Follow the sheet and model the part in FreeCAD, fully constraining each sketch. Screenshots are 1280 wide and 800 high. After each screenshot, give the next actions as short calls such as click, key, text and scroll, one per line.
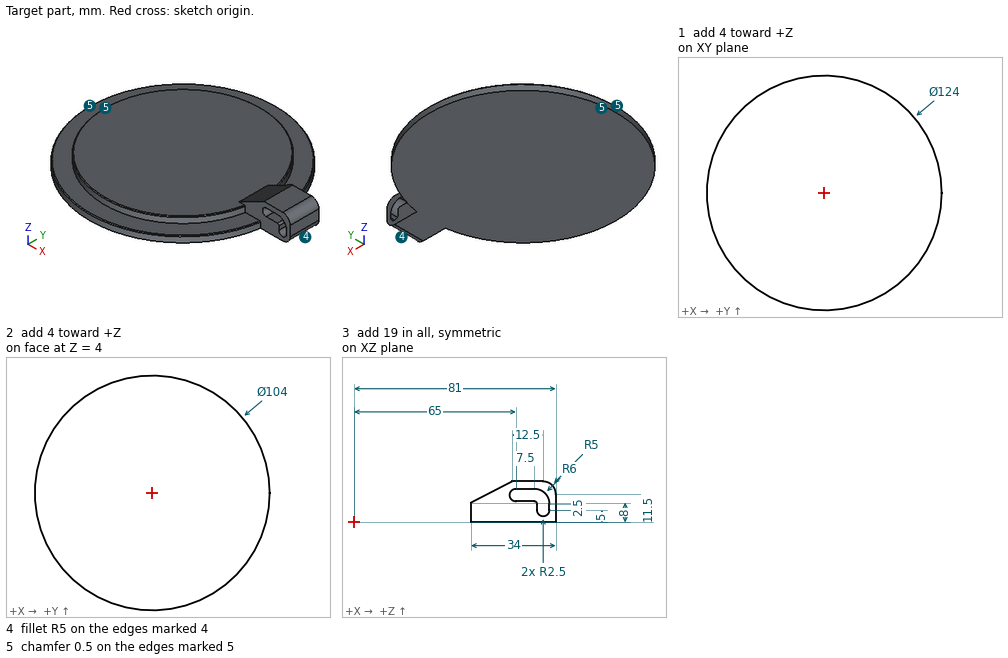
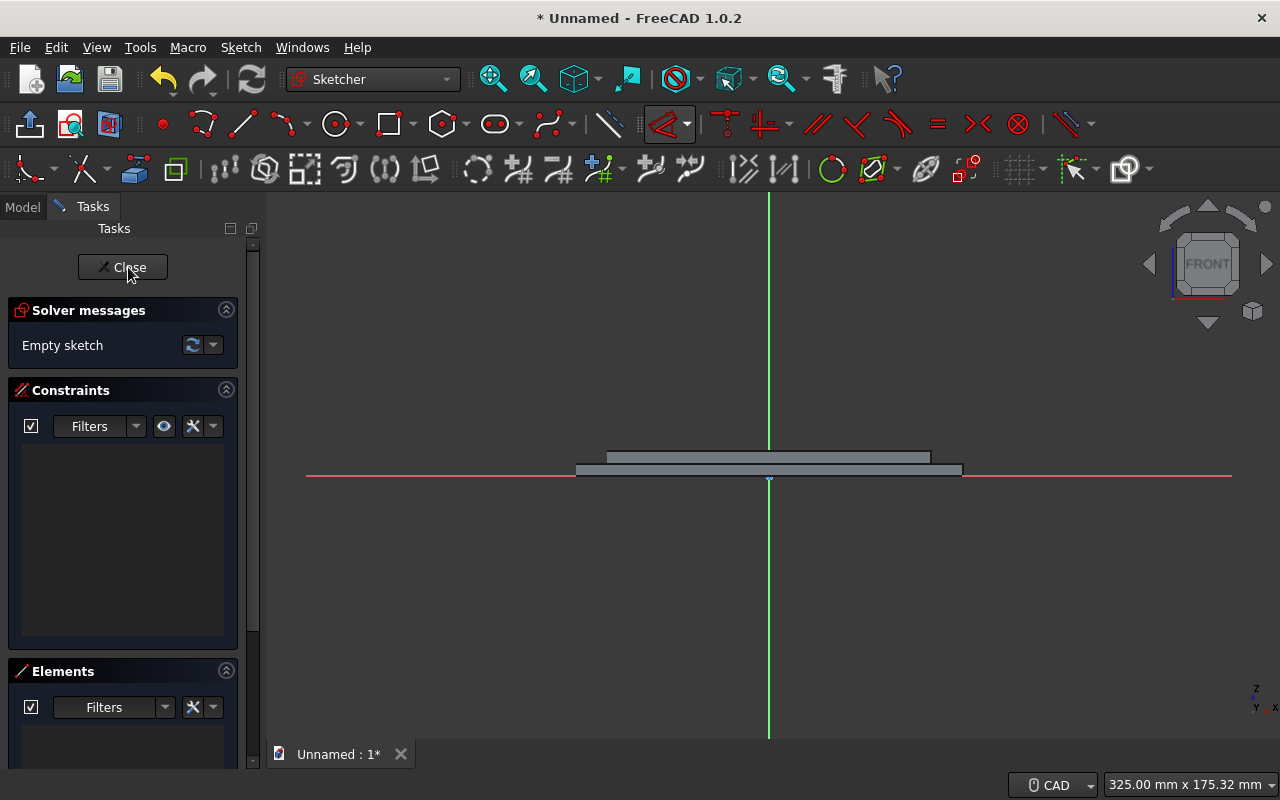
click(110, 124)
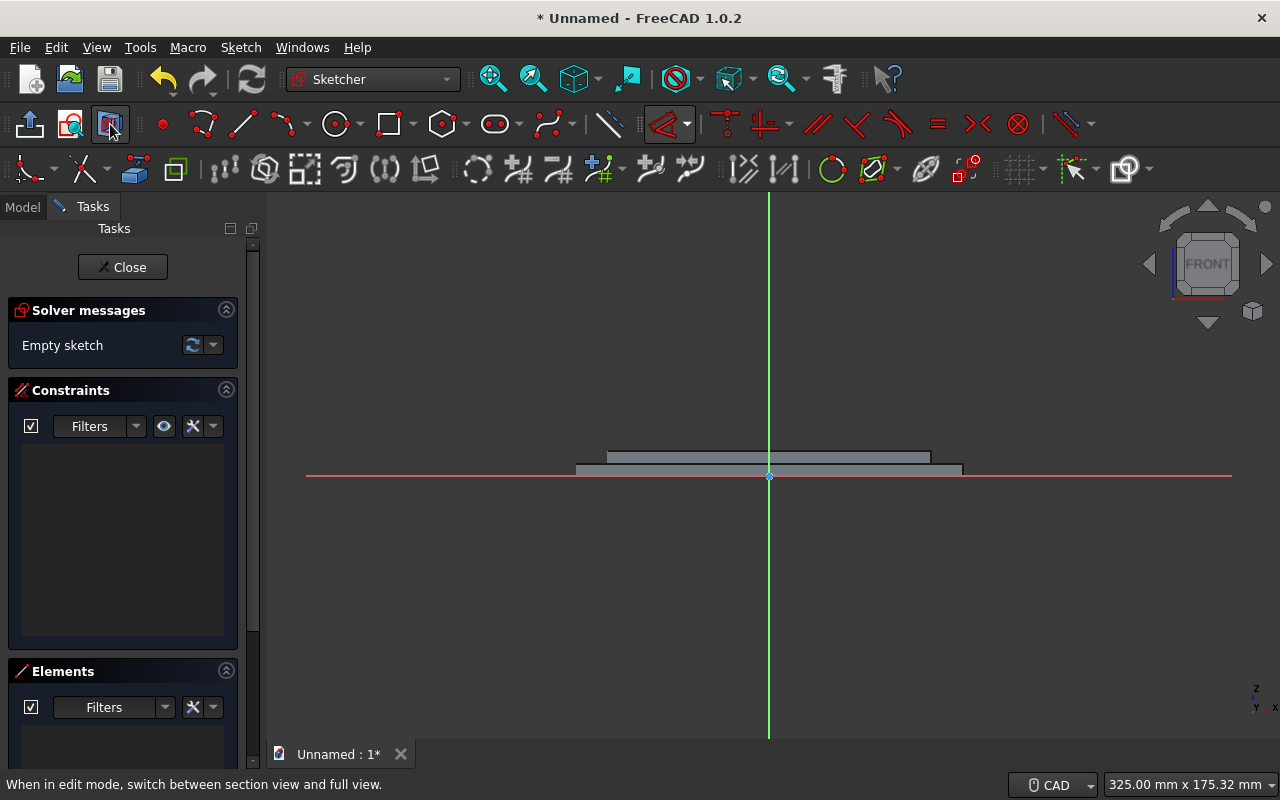
scroll(1051, 438, up, 4)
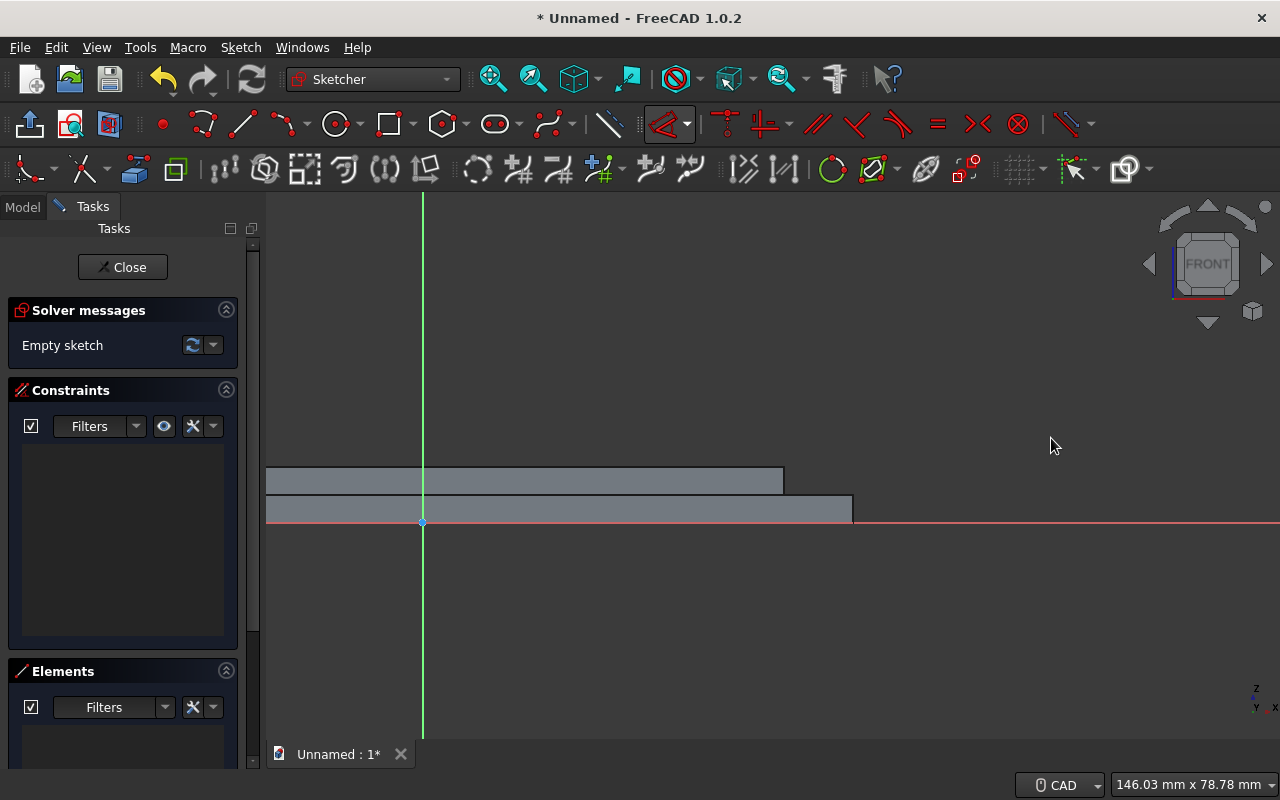
click(204, 124)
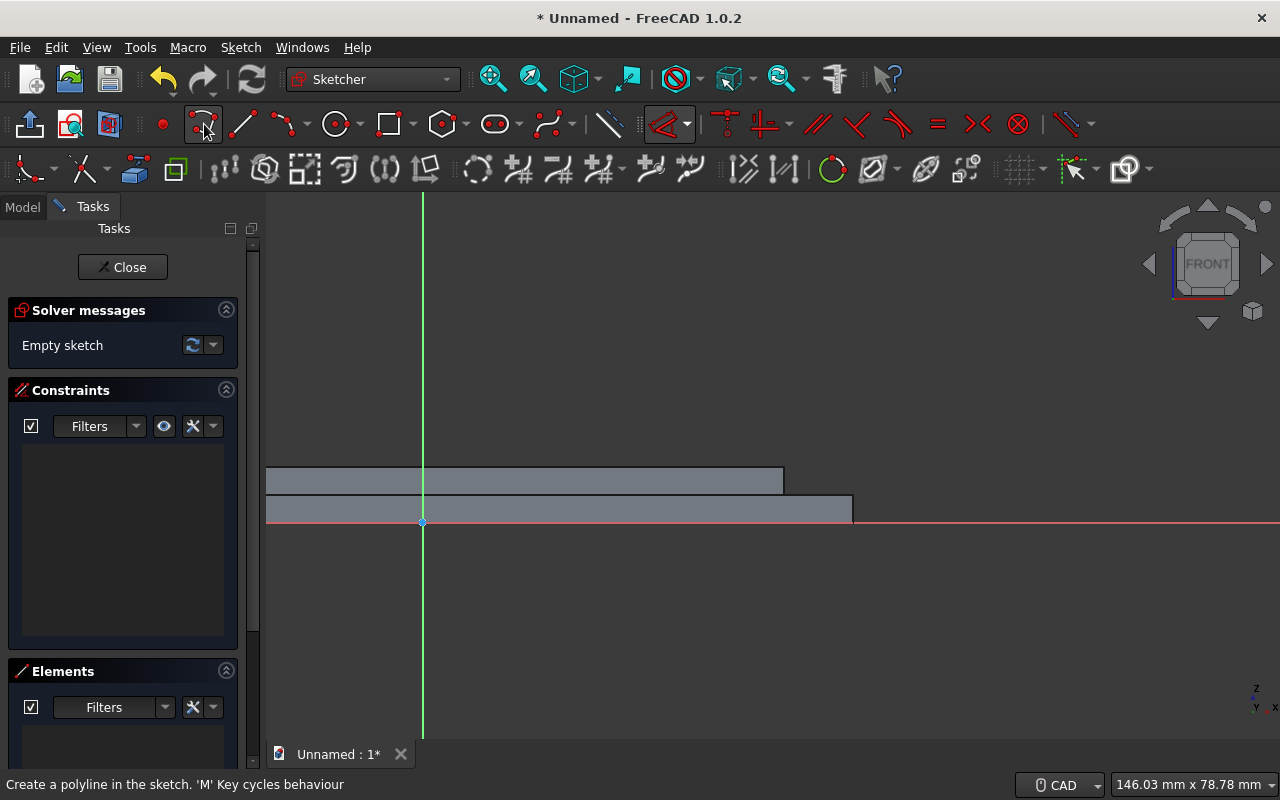
click(985, 443)
click(985, 523)
click(749, 514)
click(749, 467)
click(864, 408)
click(951, 408)
right_click(951, 408)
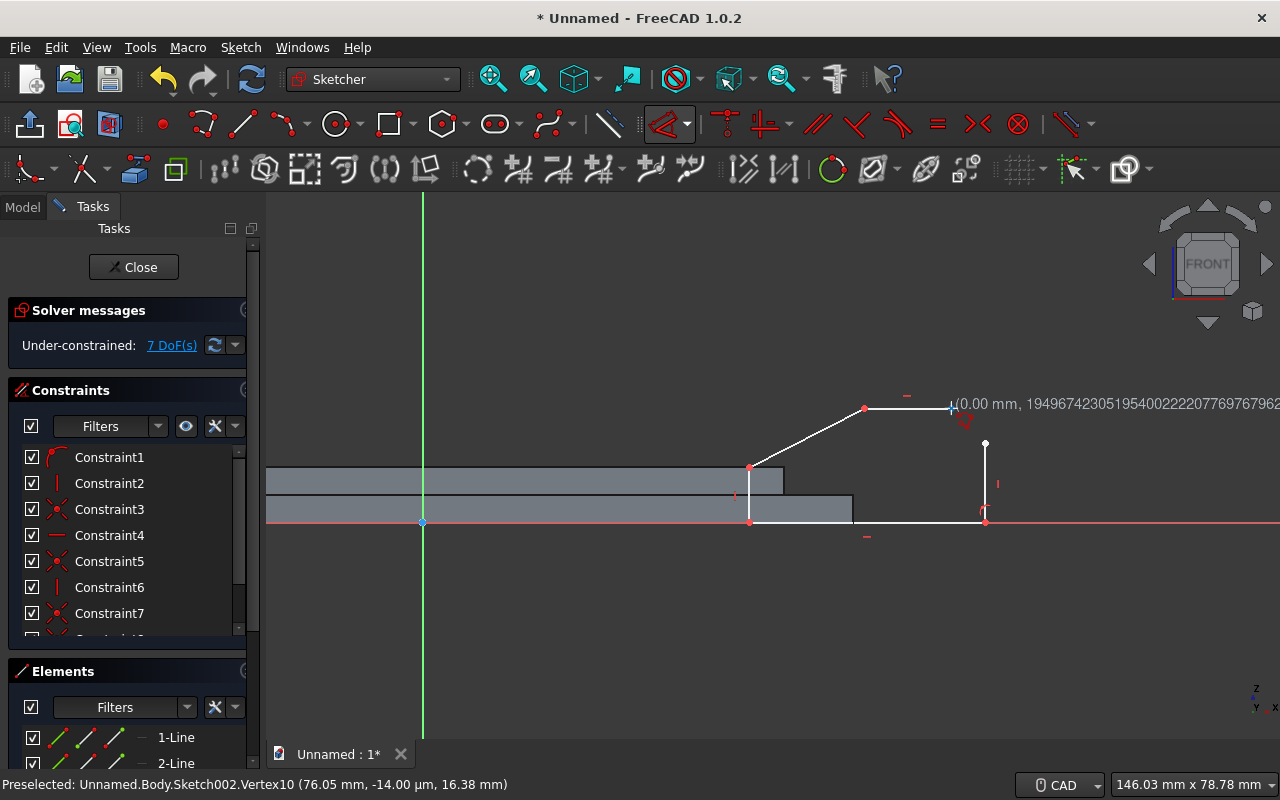
click(284, 124)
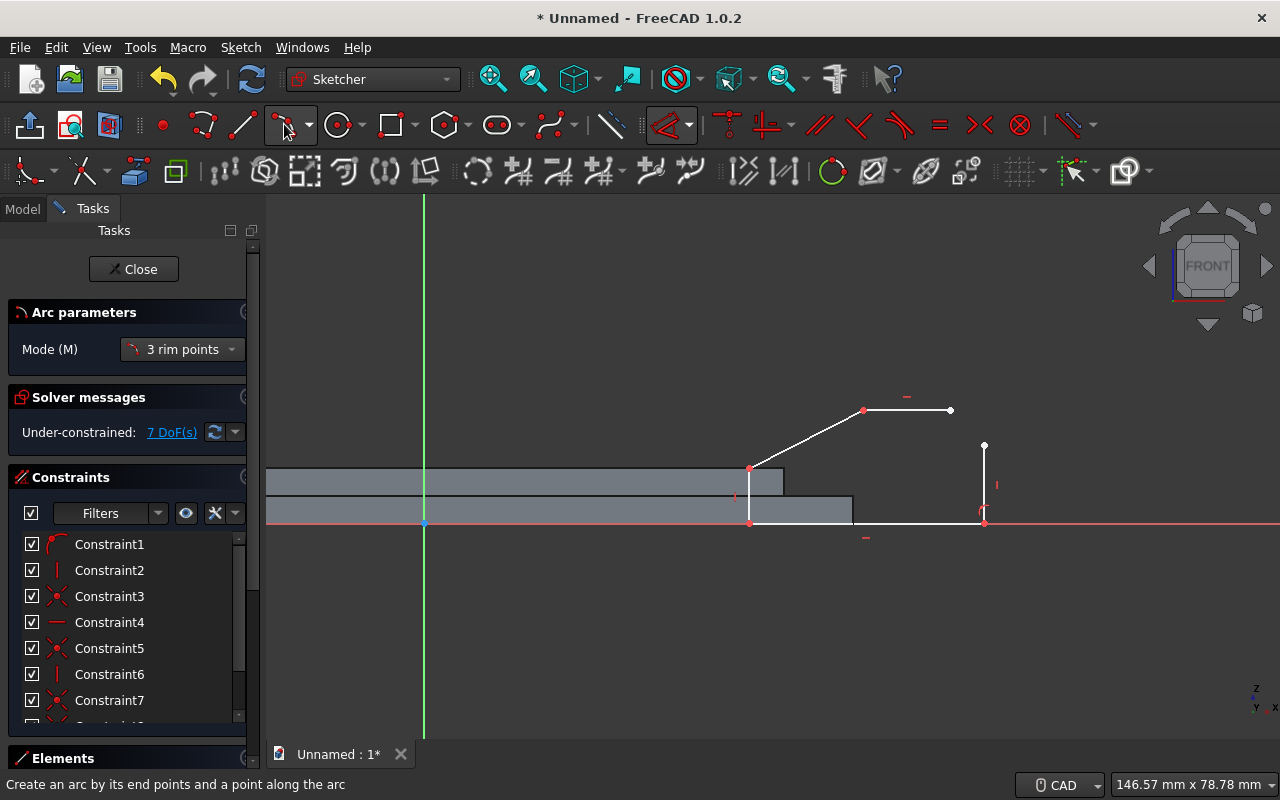
click(950, 410)
click(984, 445)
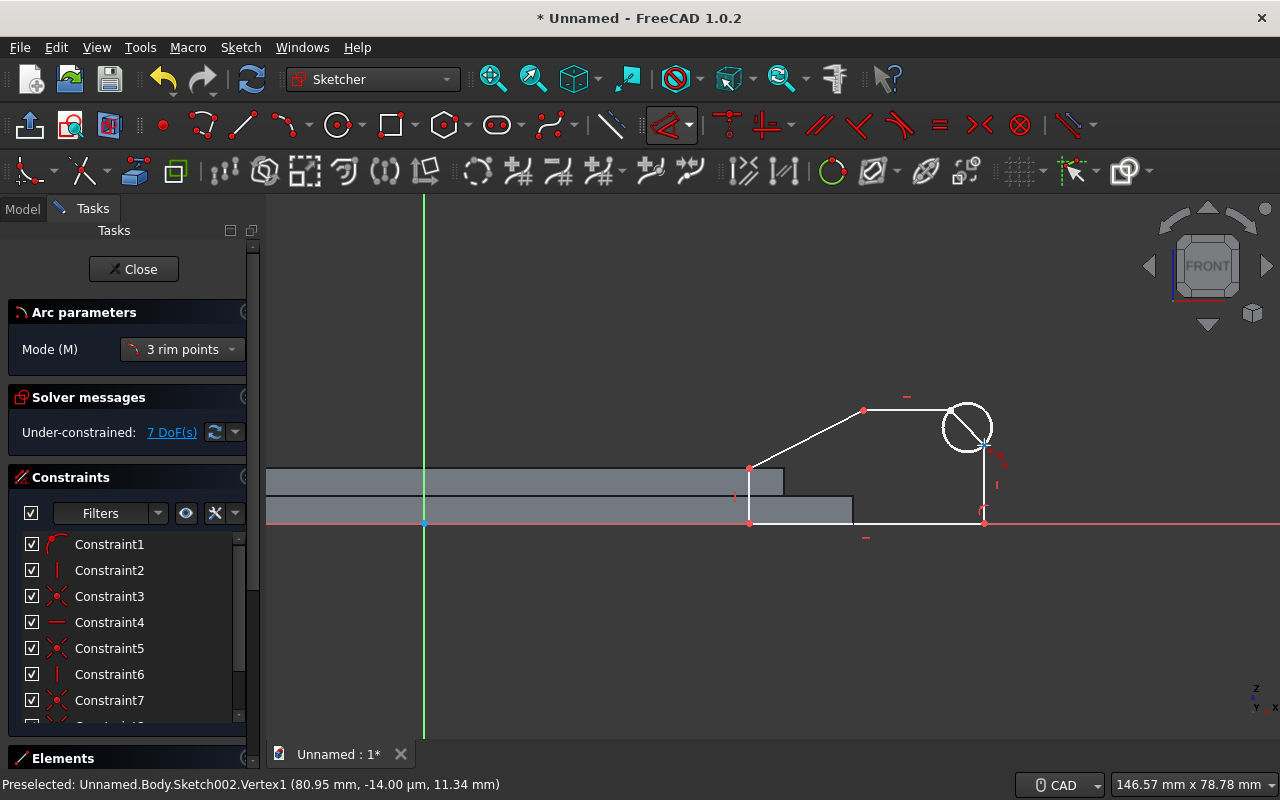
scroll(974, 419, up, 3)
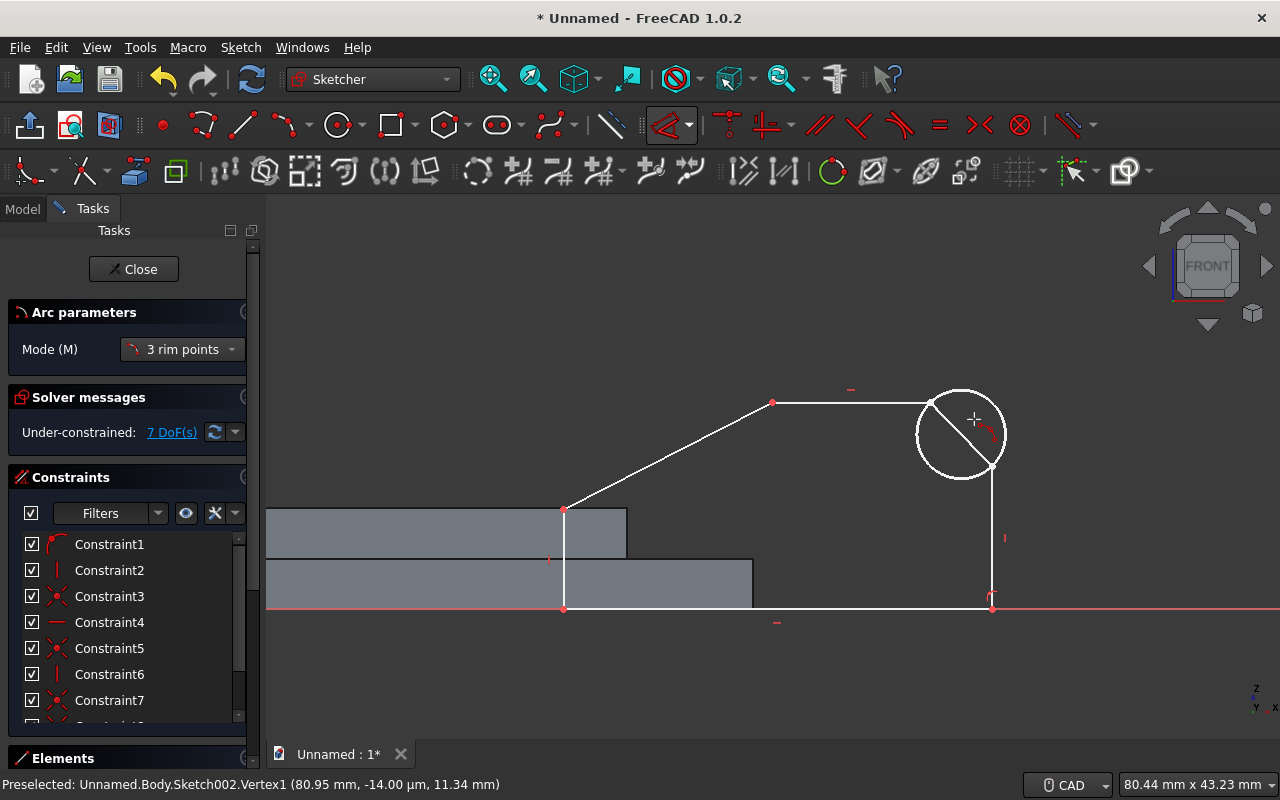
click(974, 420)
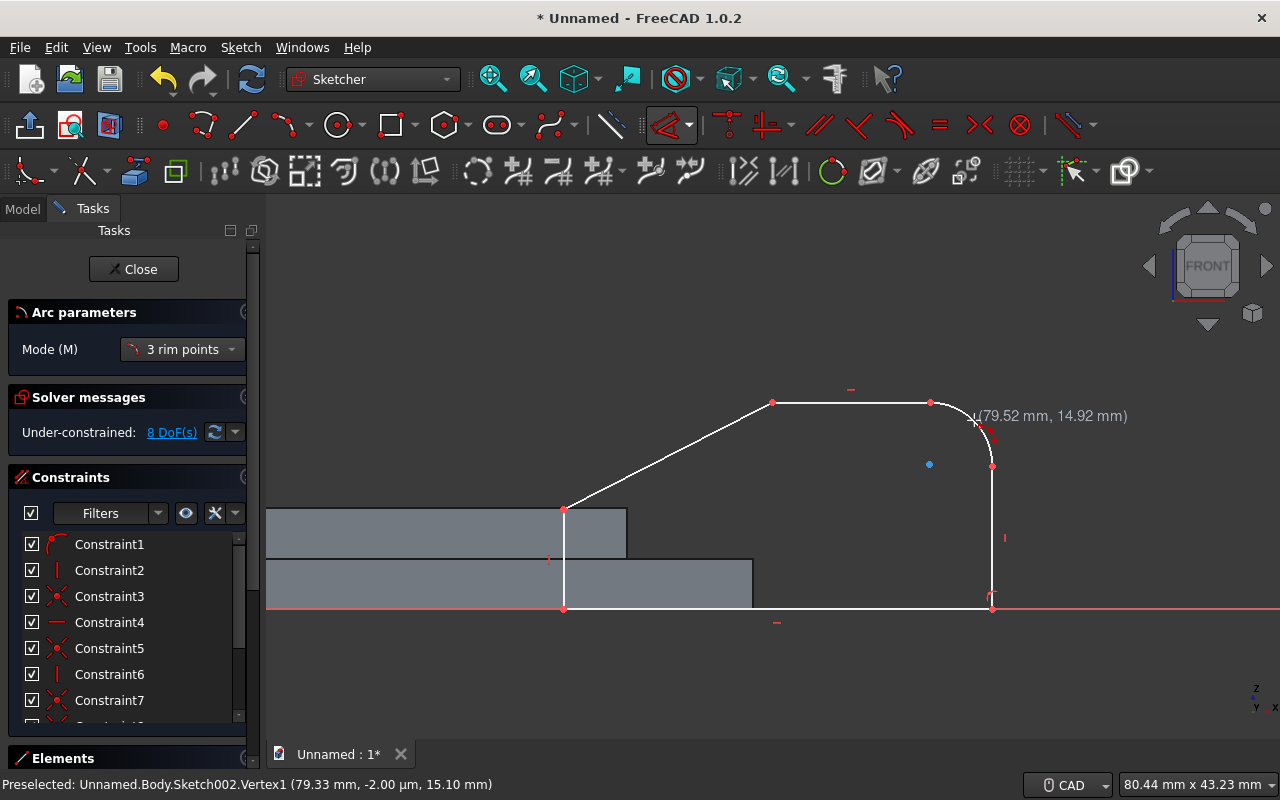
key(g)
key(l)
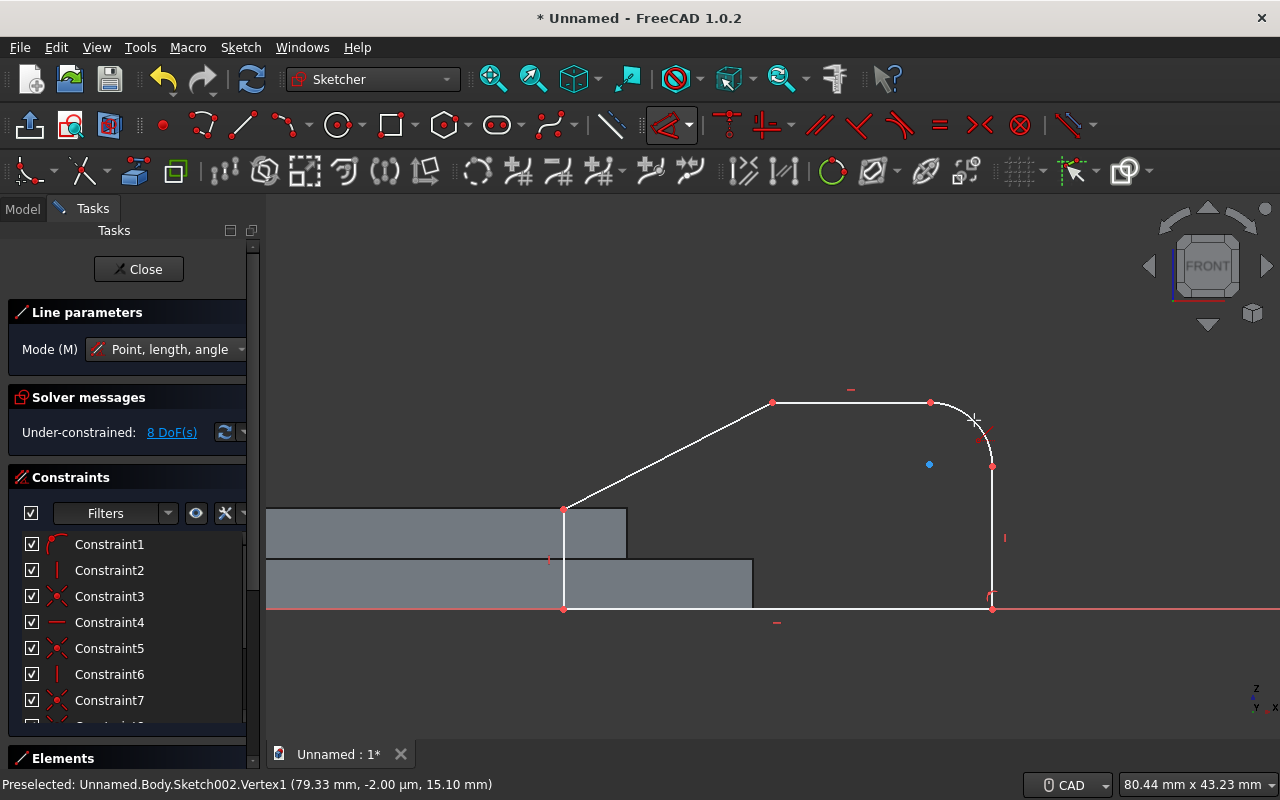
click(961, 546)
click(961, 515)